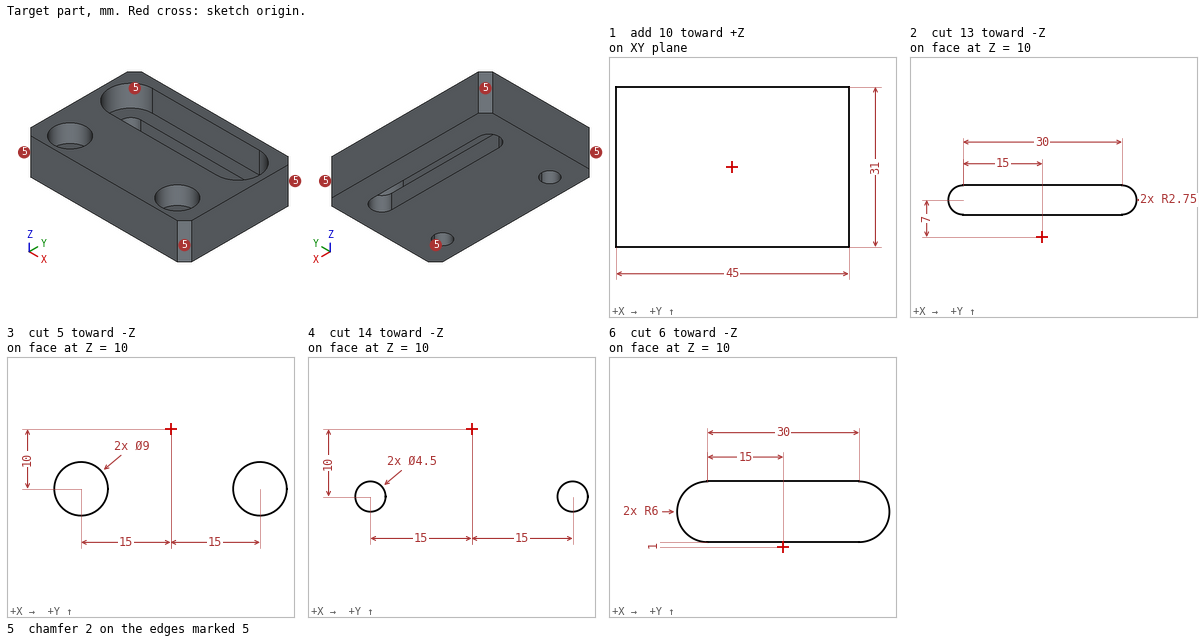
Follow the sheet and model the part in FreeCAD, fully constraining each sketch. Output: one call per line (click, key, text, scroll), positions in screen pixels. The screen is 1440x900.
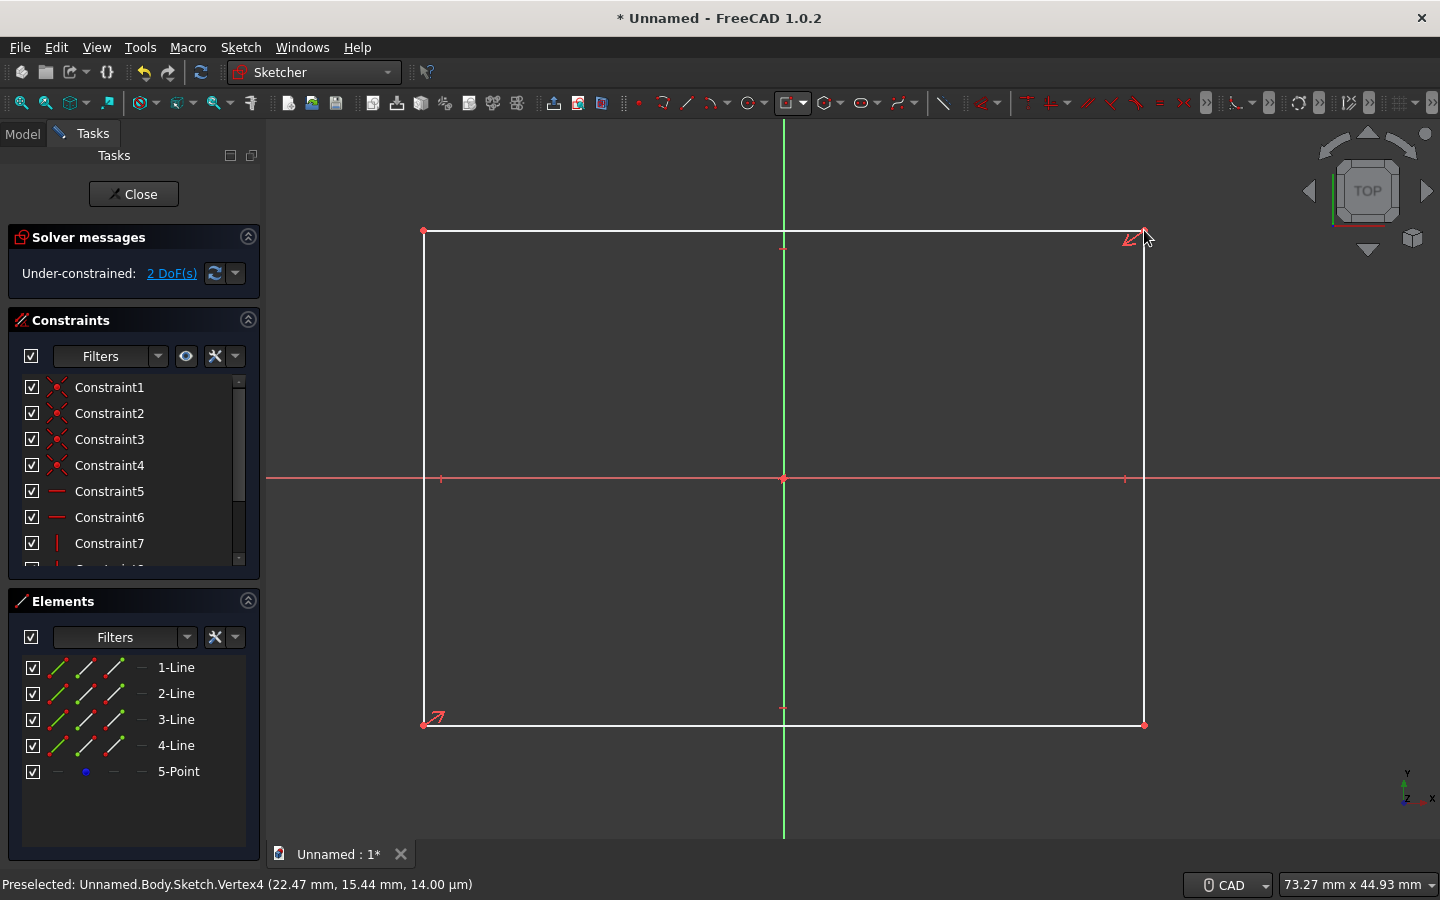
click(982, 104)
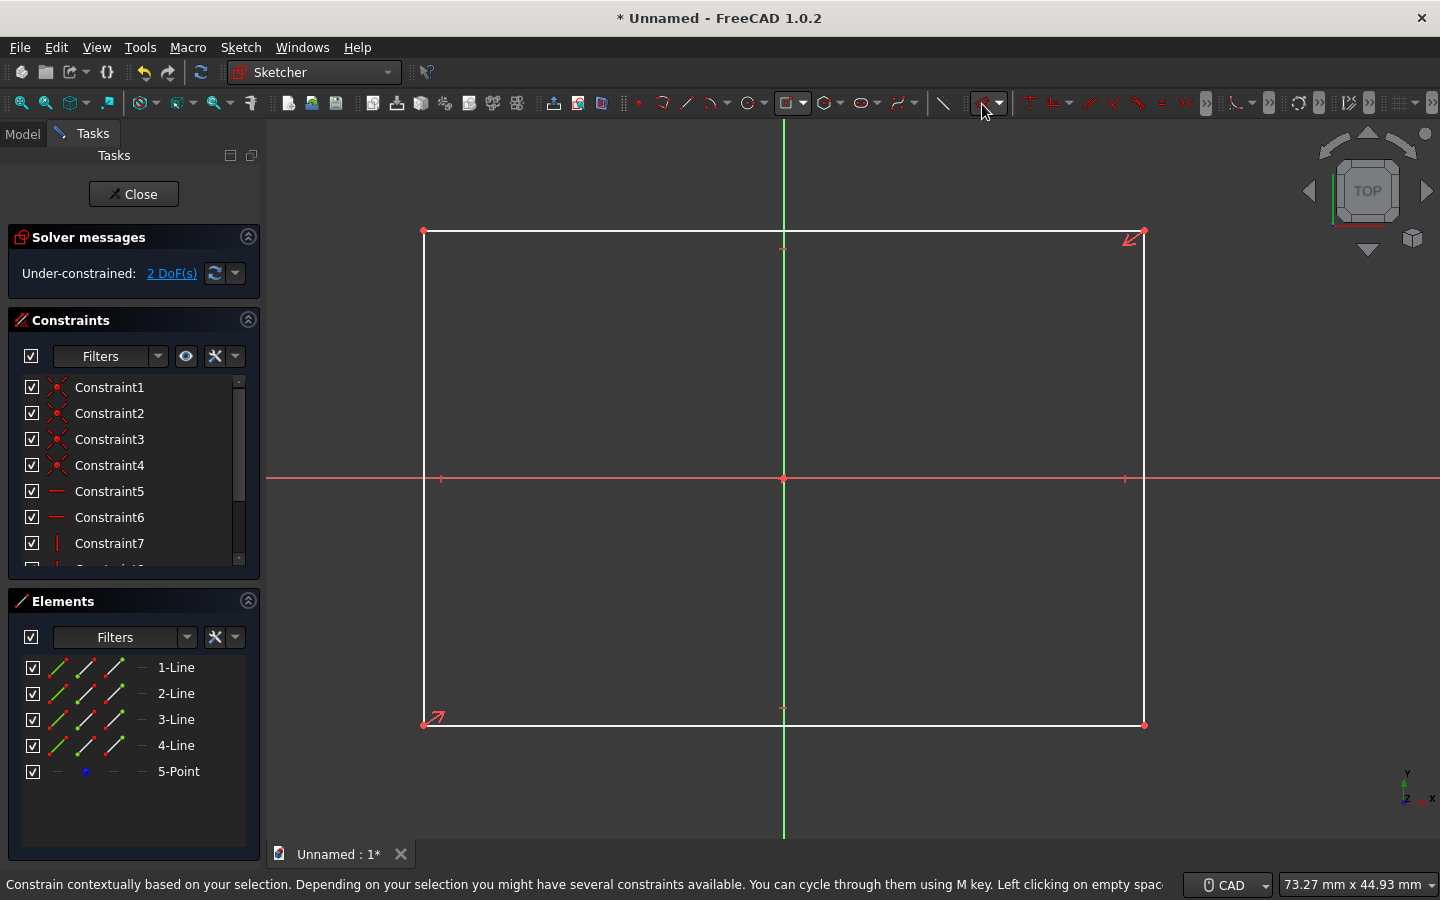
click(640, 726)
click(618, 760)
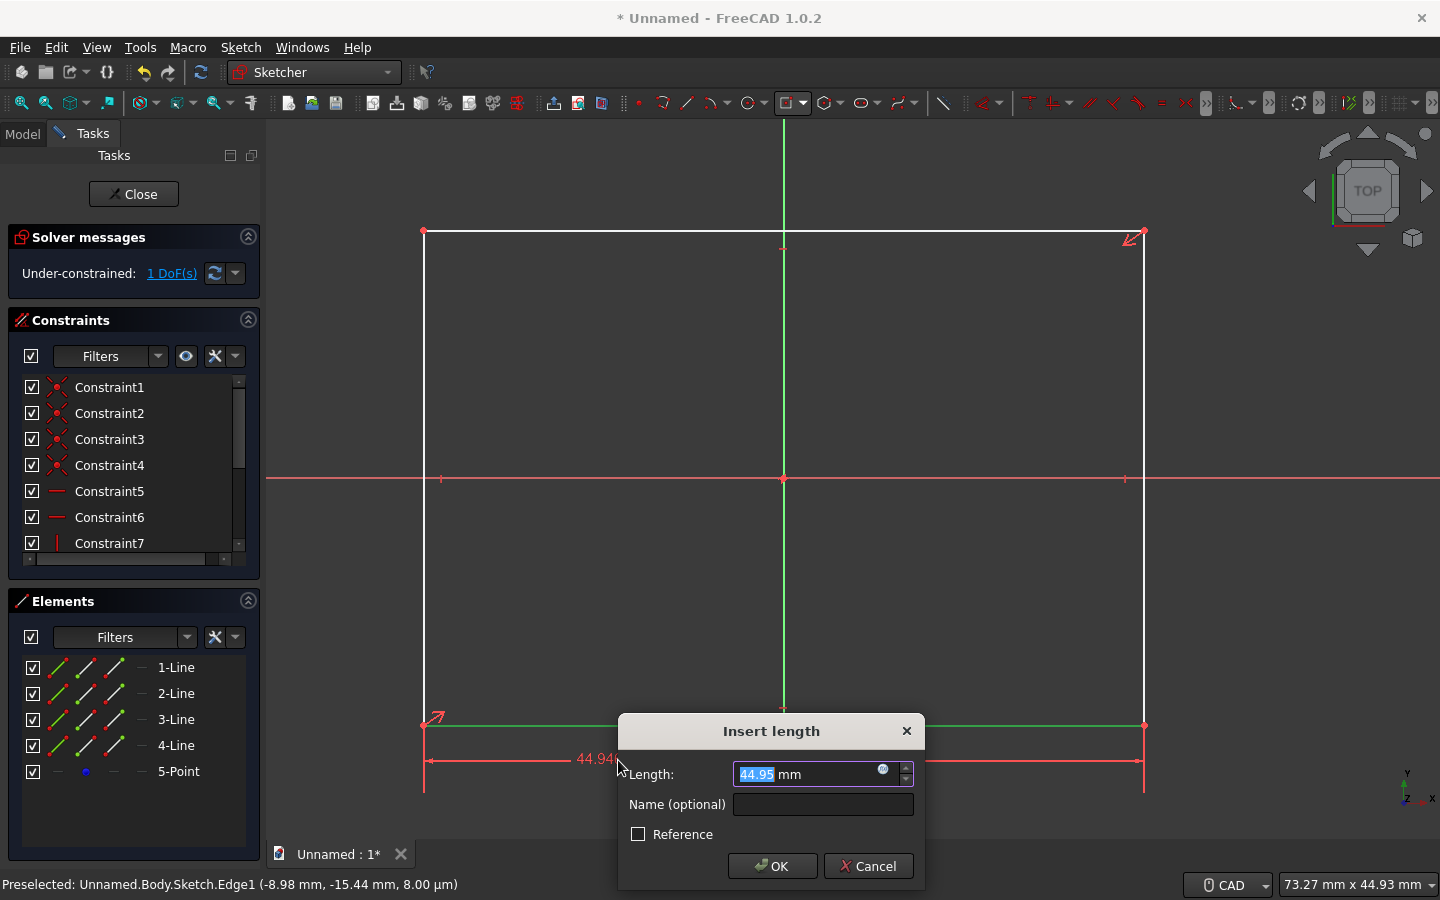
text(45)
key(Return)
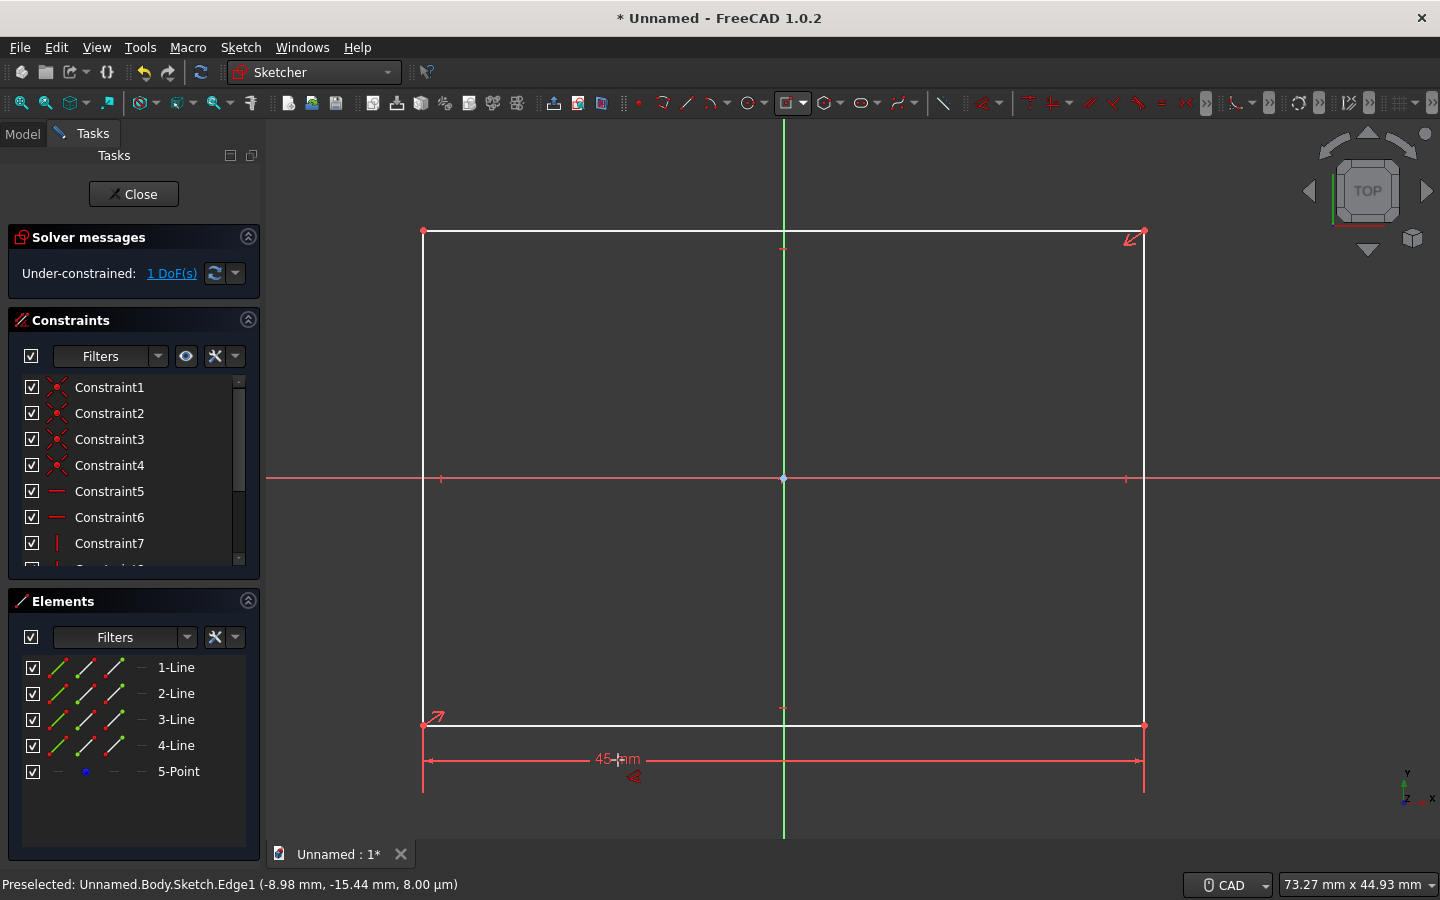
click(1144, 577)
click(1178, 365)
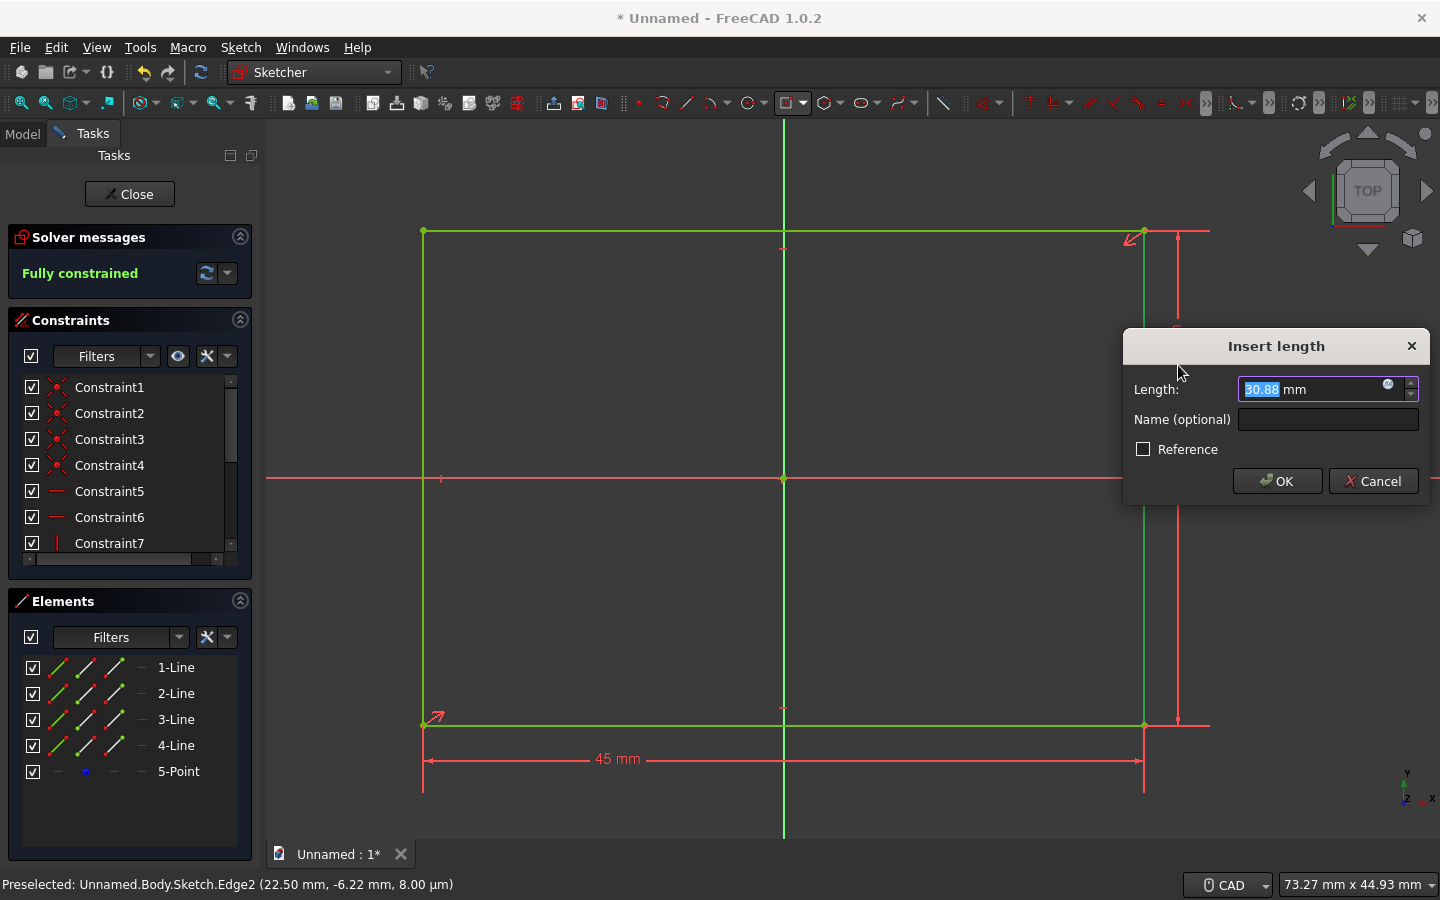
text(31)
key(Return)
key(Escape)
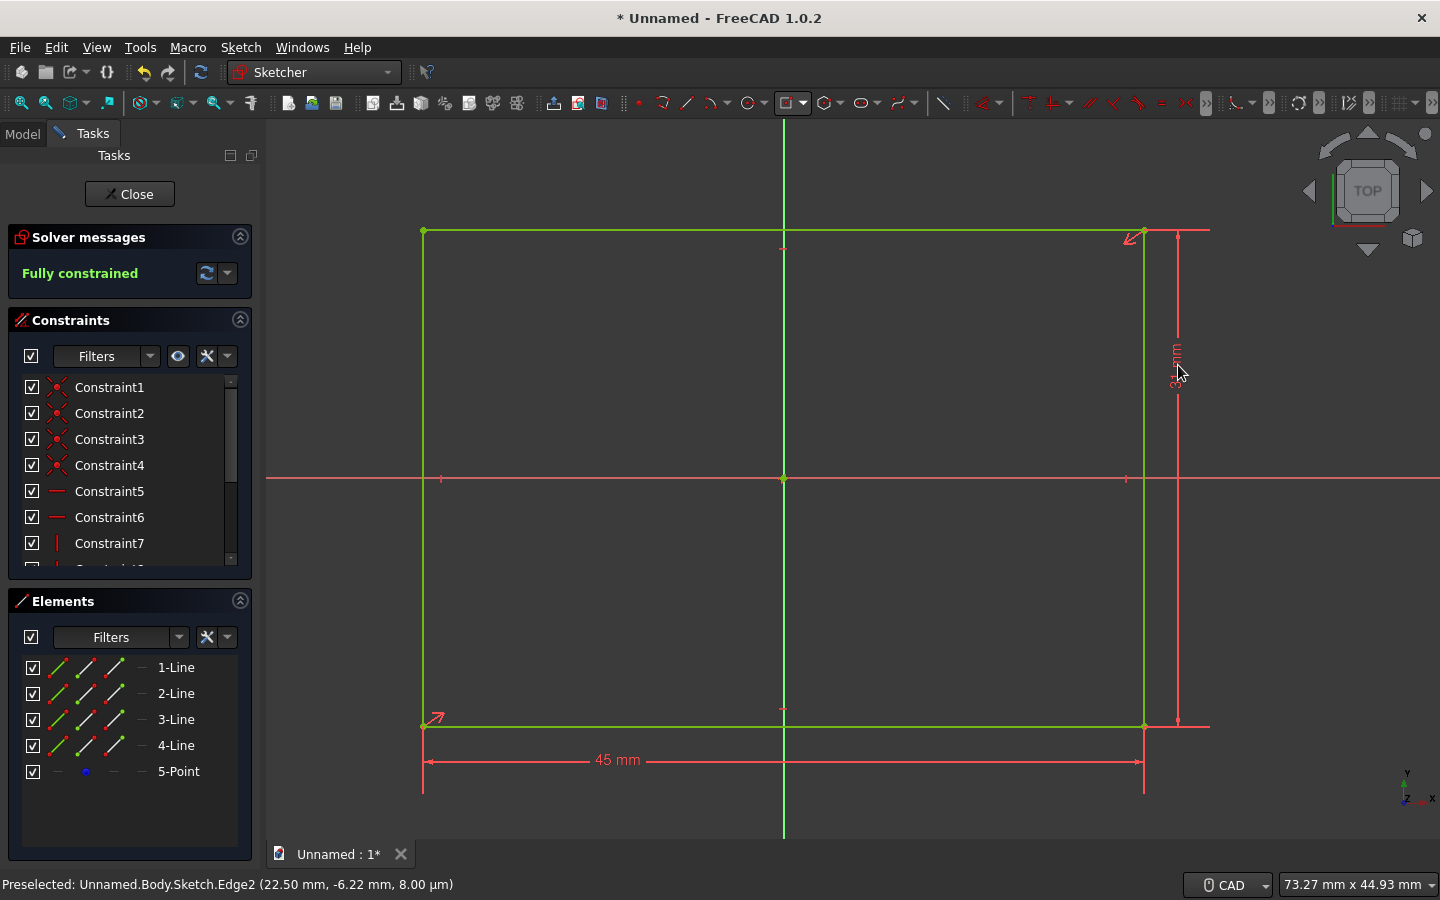
click(130, 194)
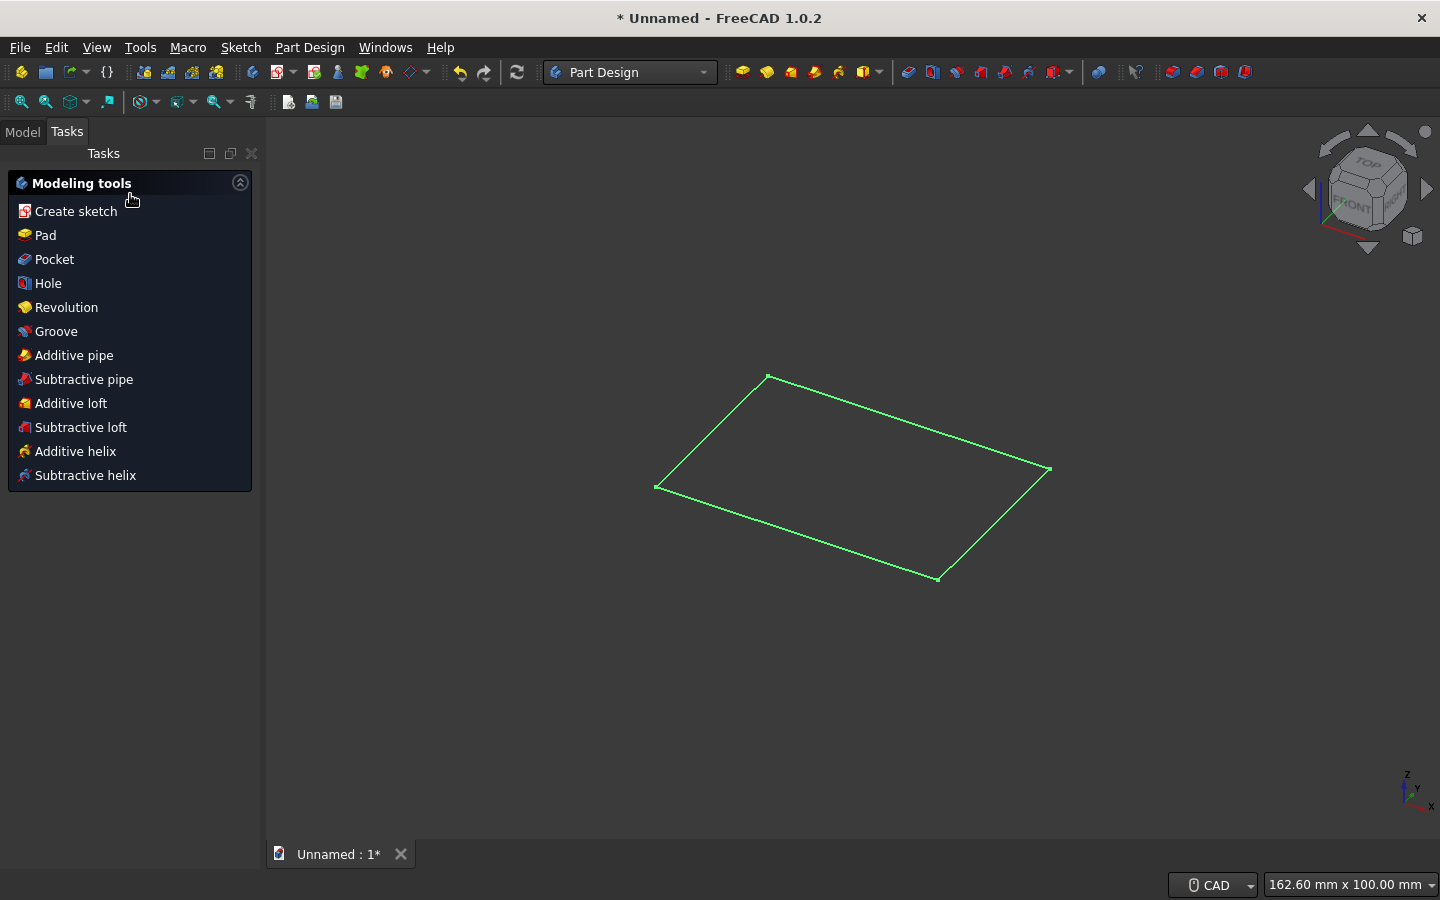
click(744, 72)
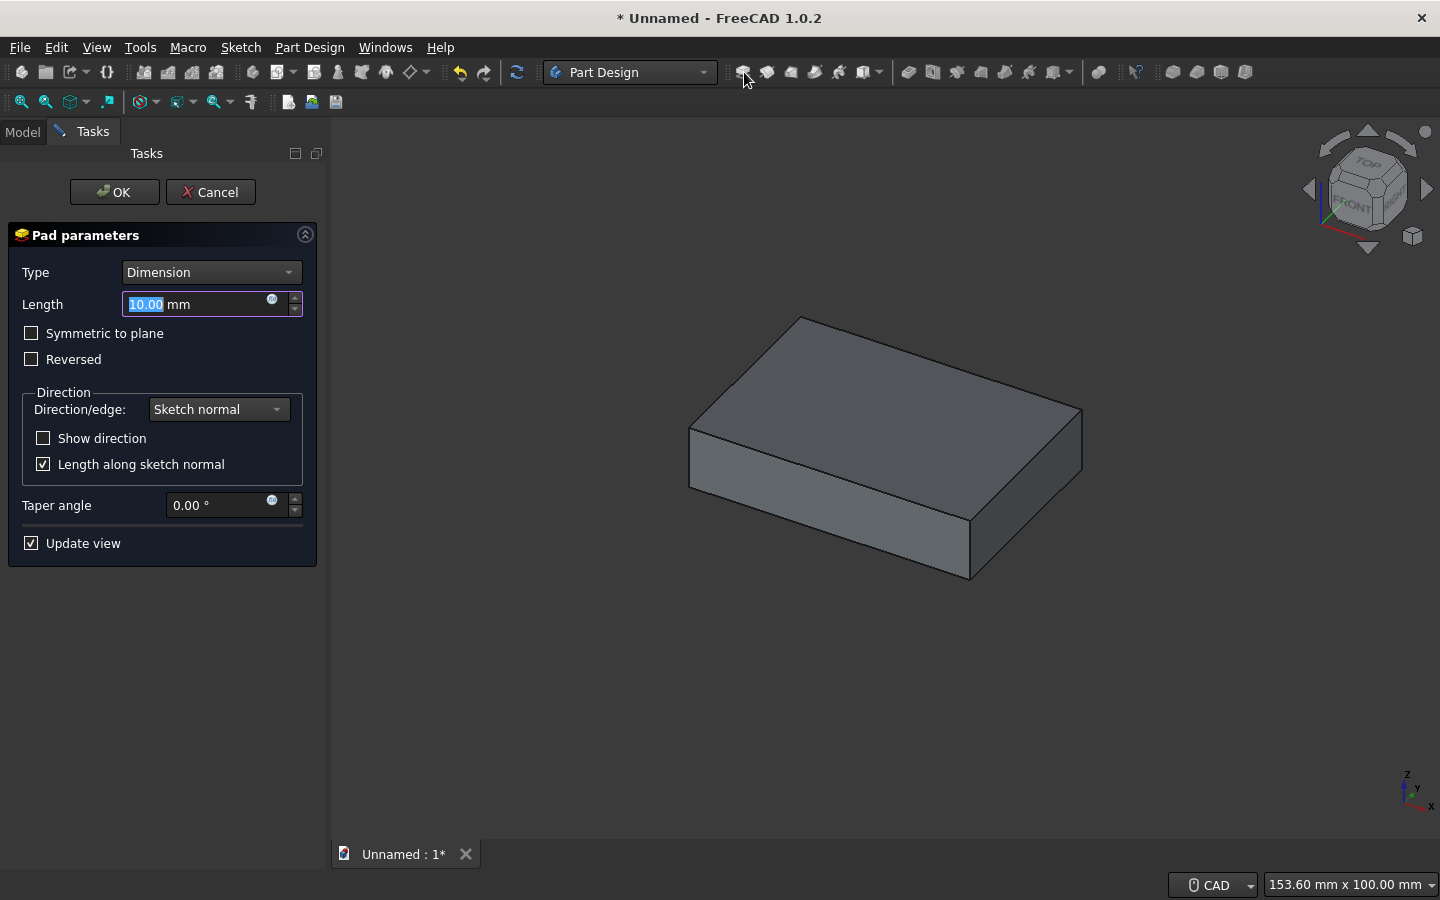
text(10)
key(Tab)